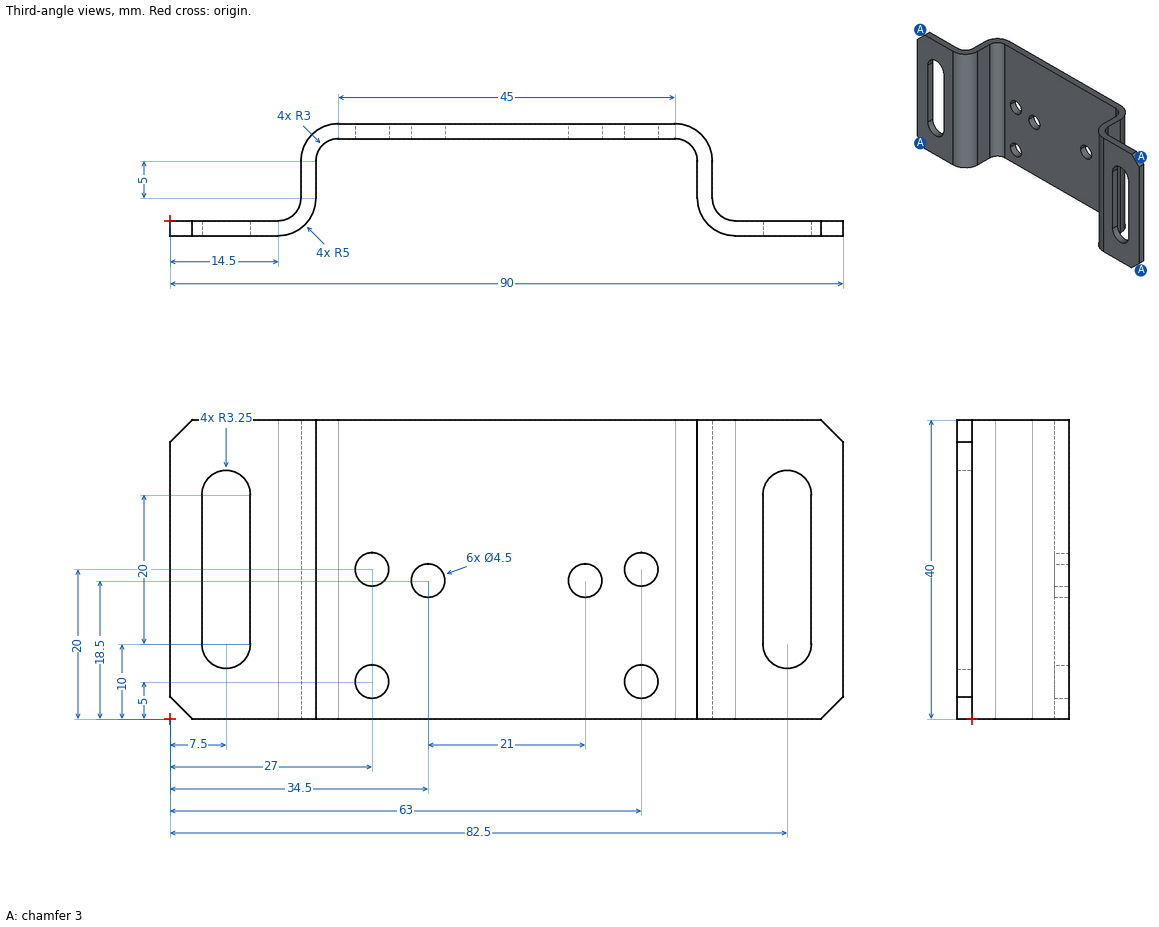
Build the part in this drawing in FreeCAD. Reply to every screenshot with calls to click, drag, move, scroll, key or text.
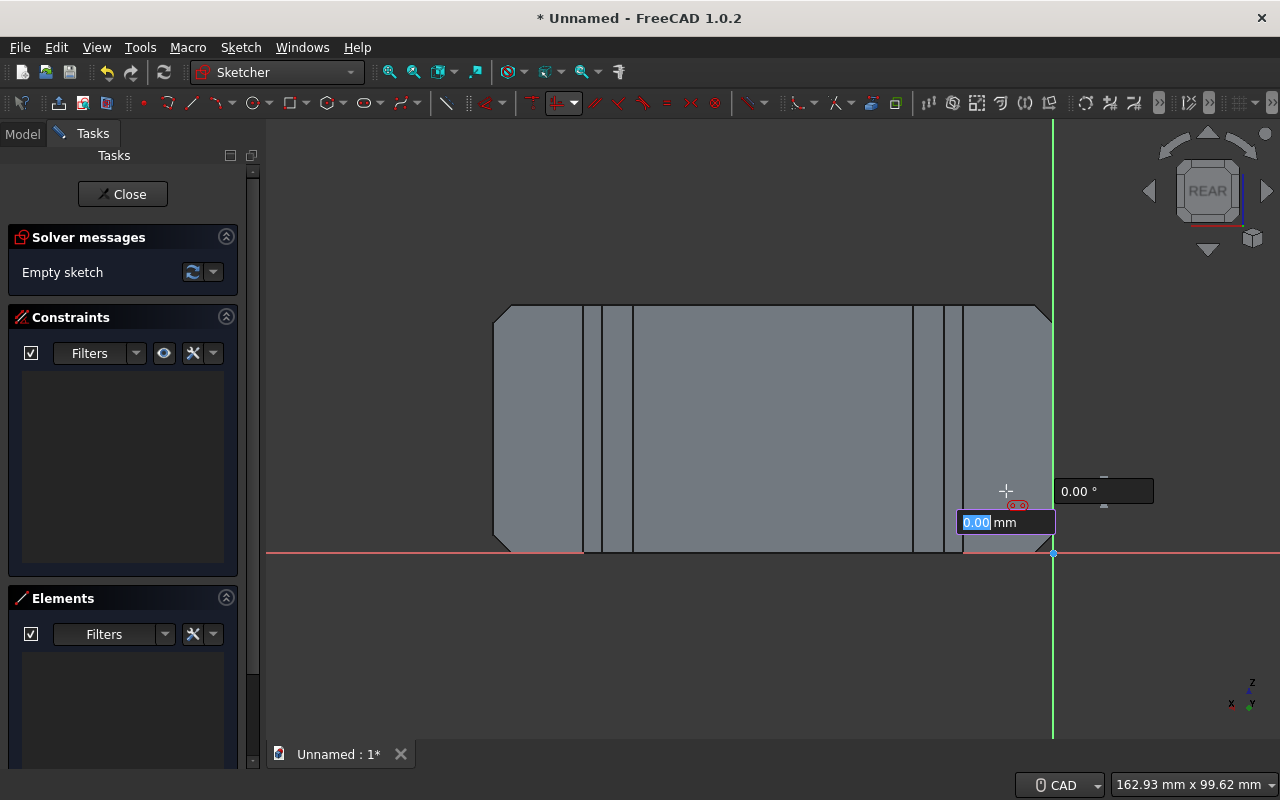
click(1006, 367)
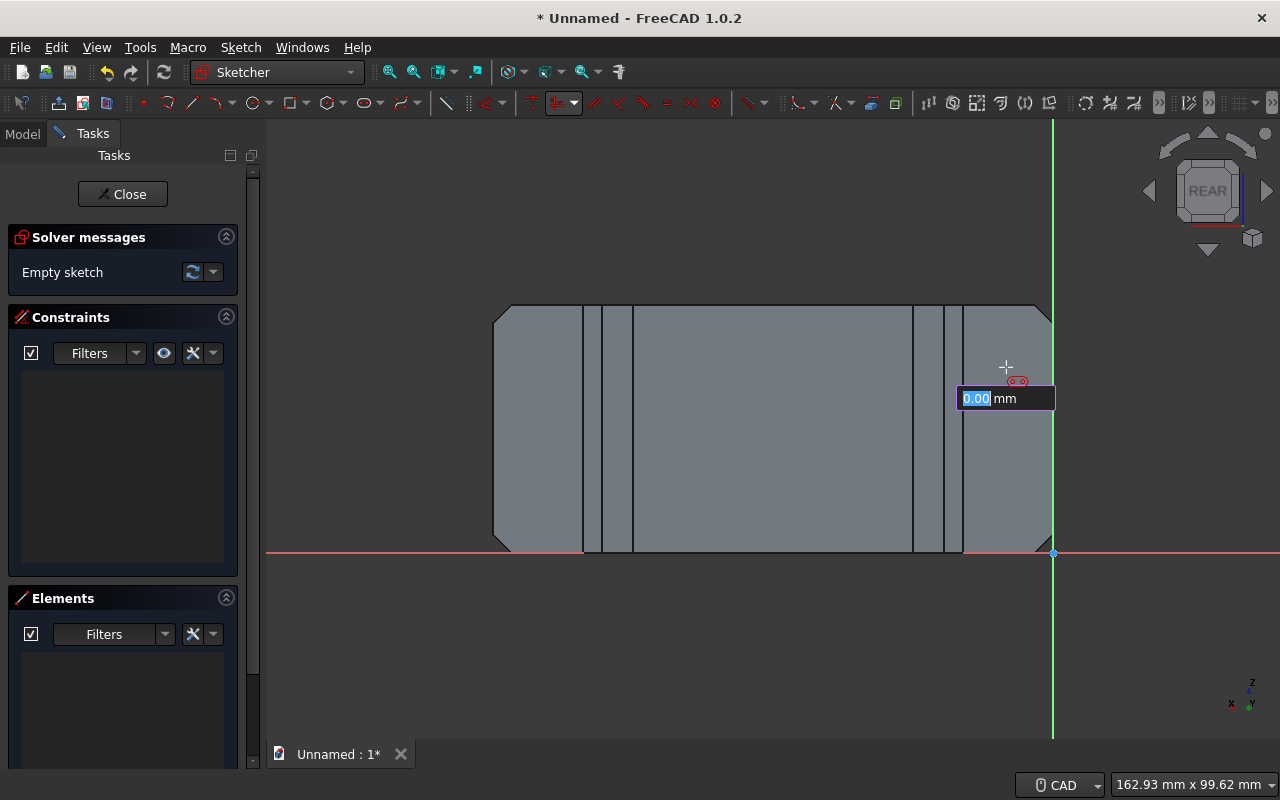
click(1027, 429)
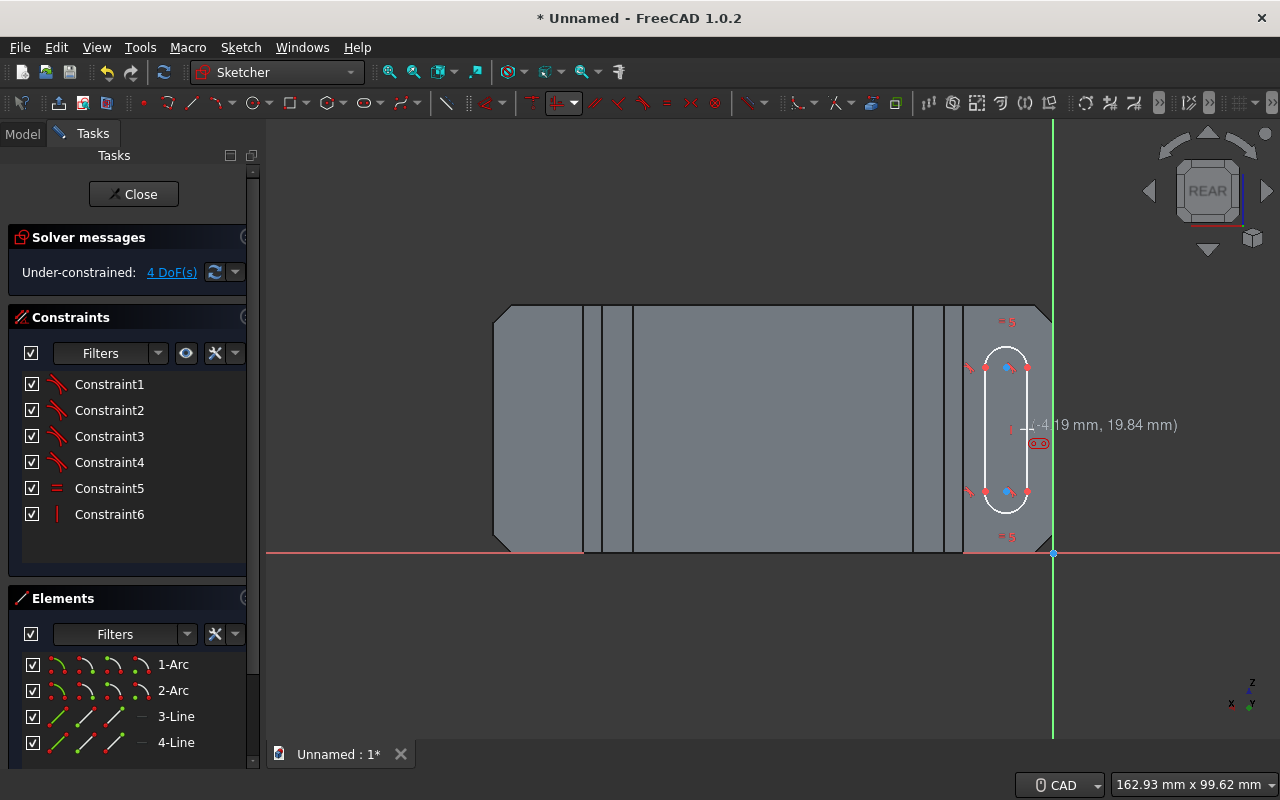
click(540, 491)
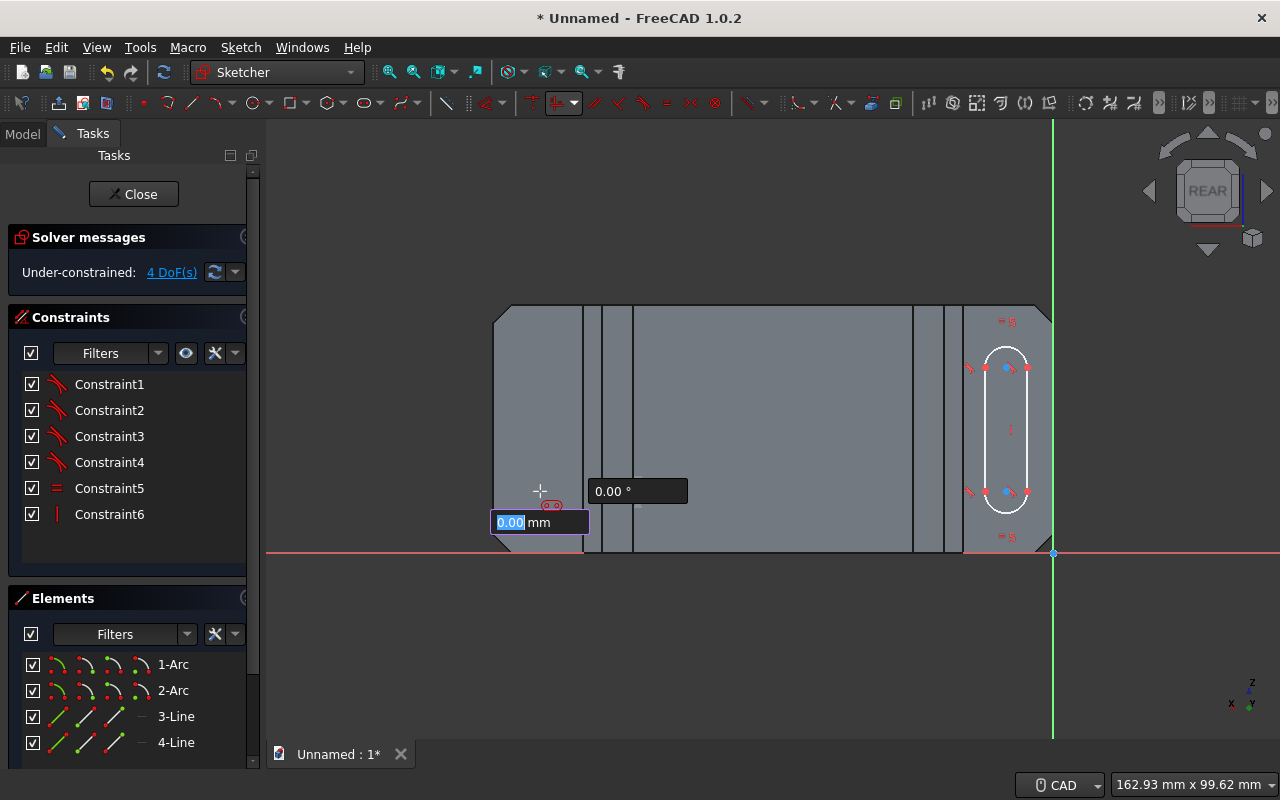
click(540, 367)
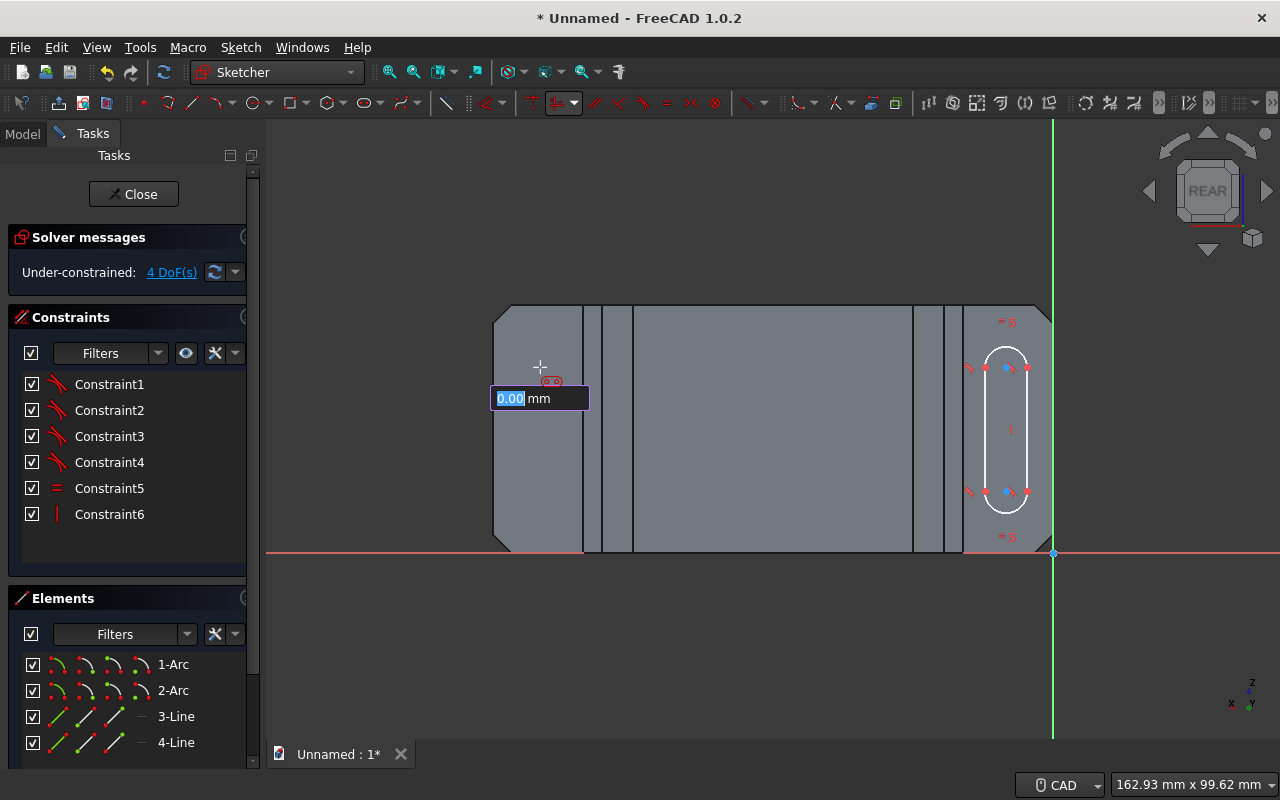
click(519, 429)
key(Escape)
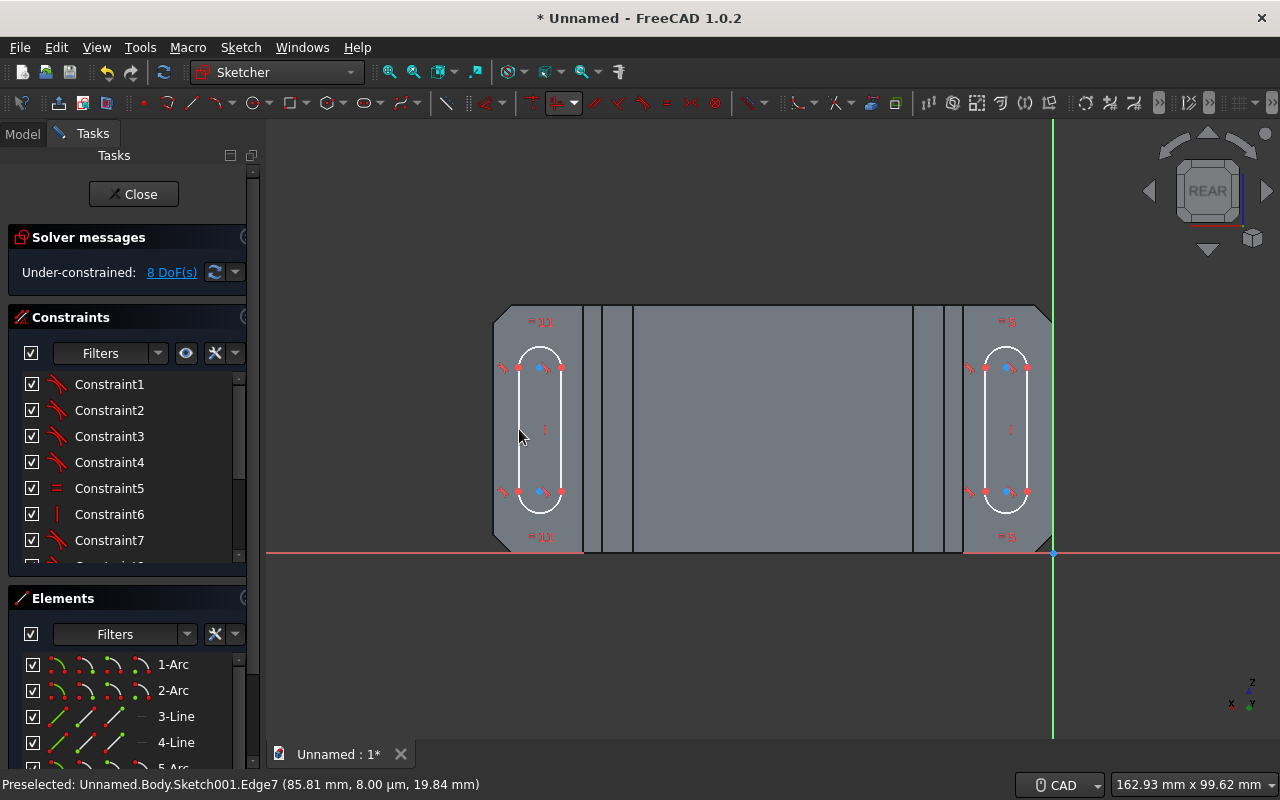
click(994, 509)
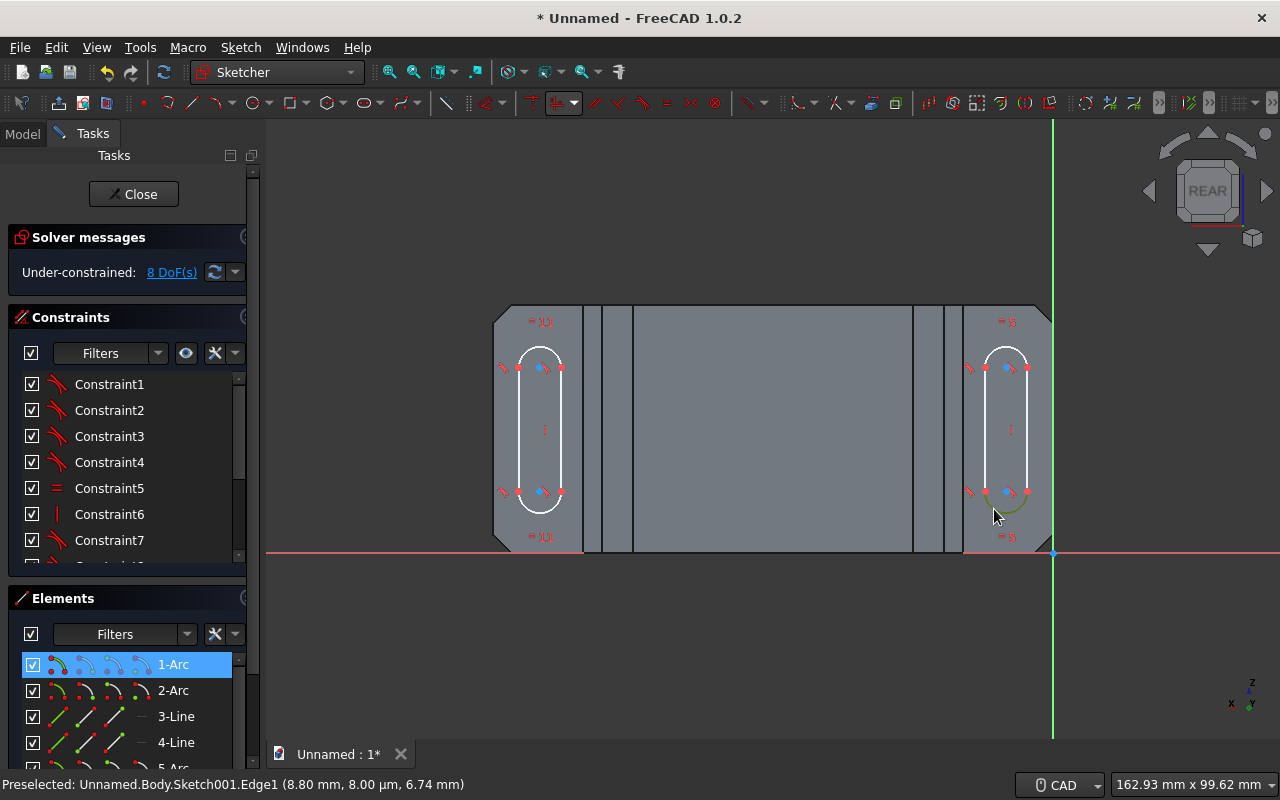
click(528, 509)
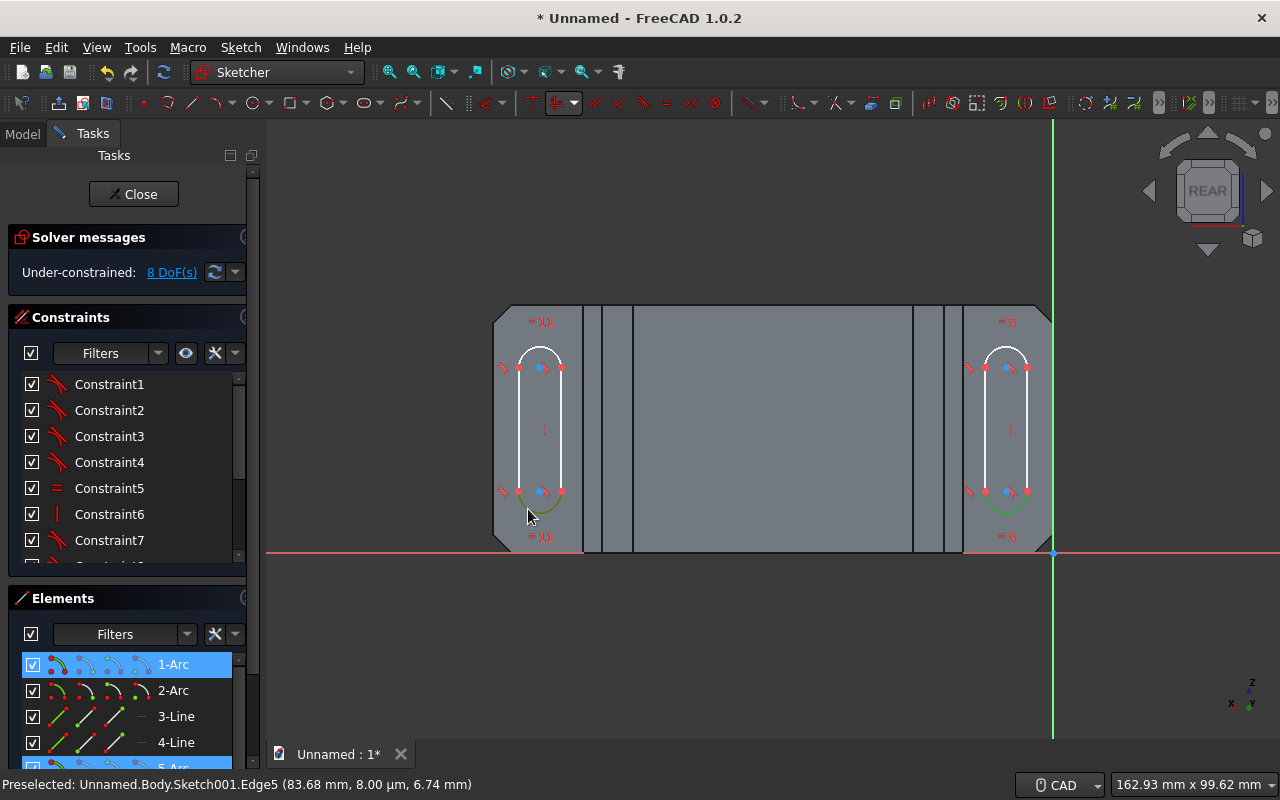
key(e)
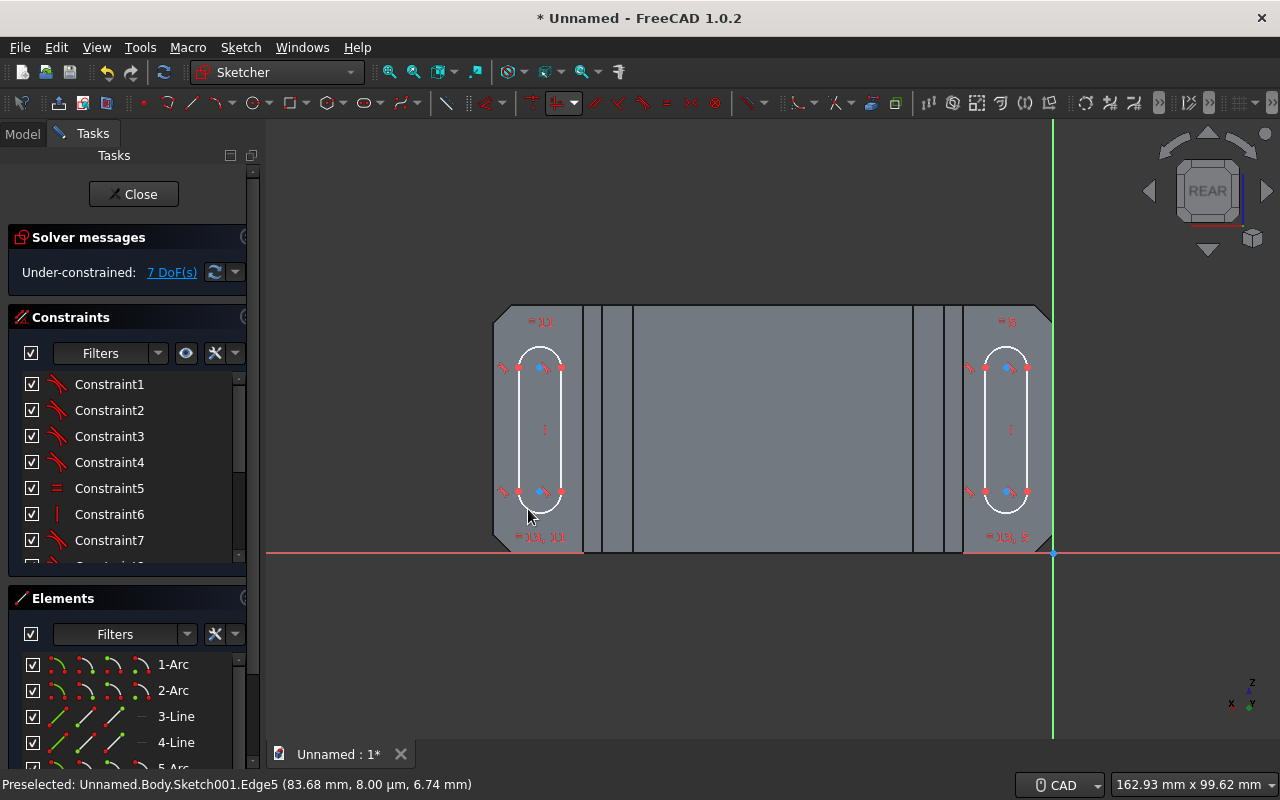
key(d)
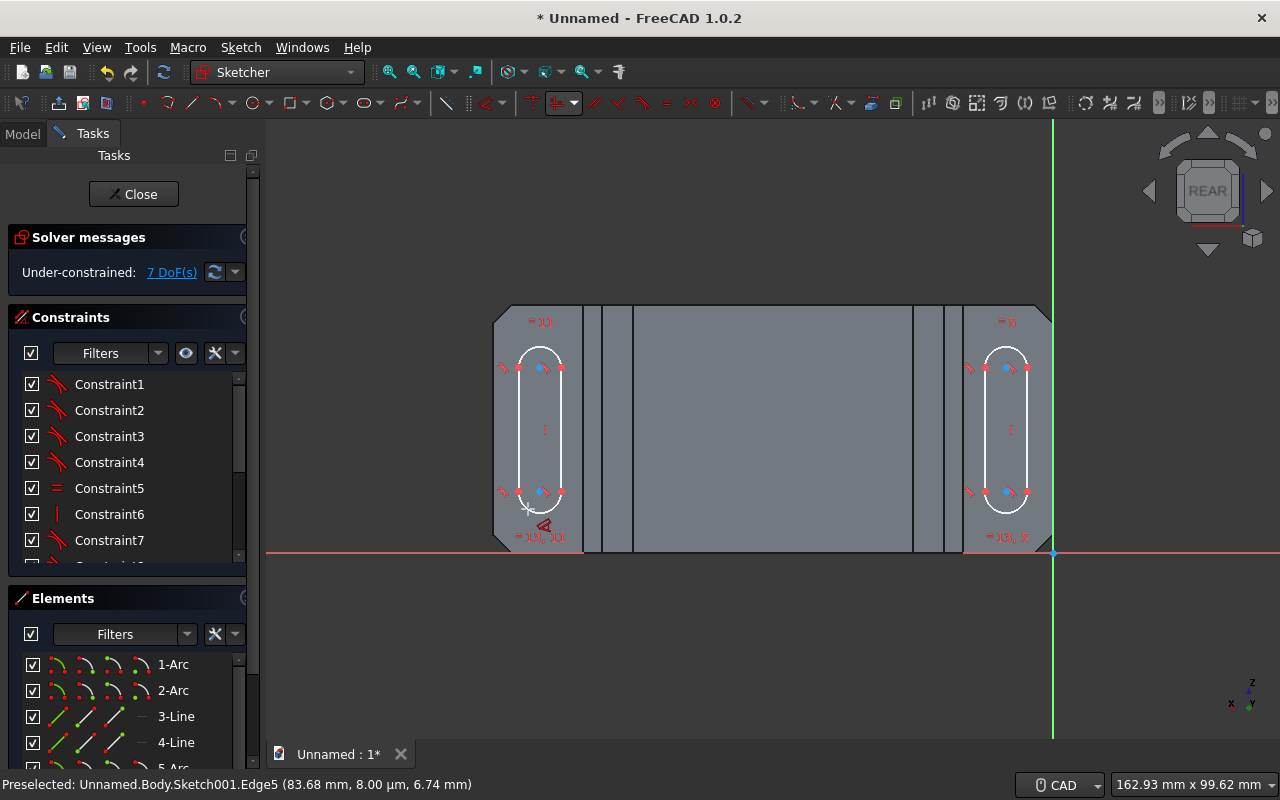
scroll(994, 509, up, 4)